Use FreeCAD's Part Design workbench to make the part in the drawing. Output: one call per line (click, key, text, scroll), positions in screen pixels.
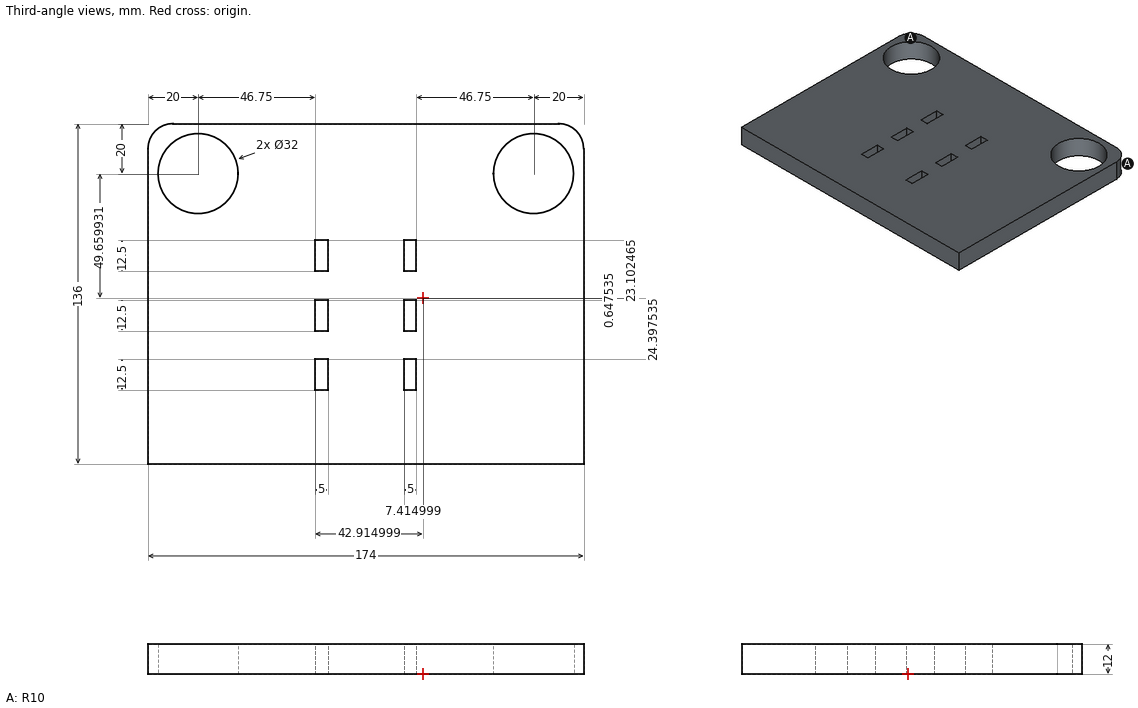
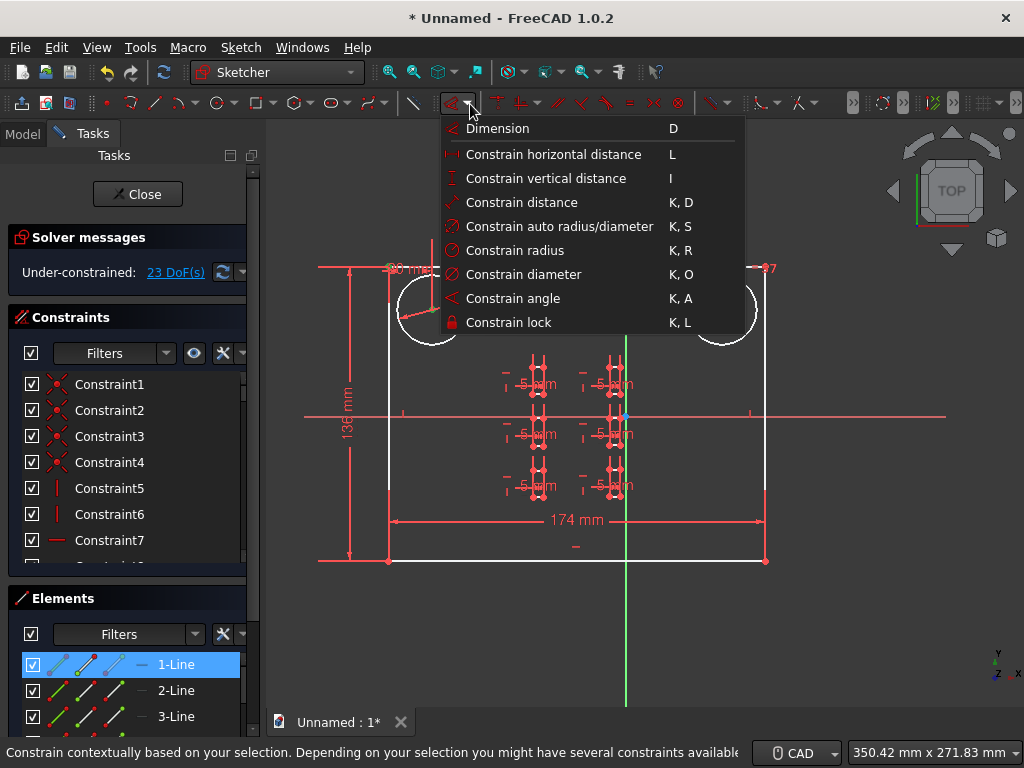
click(593, 178)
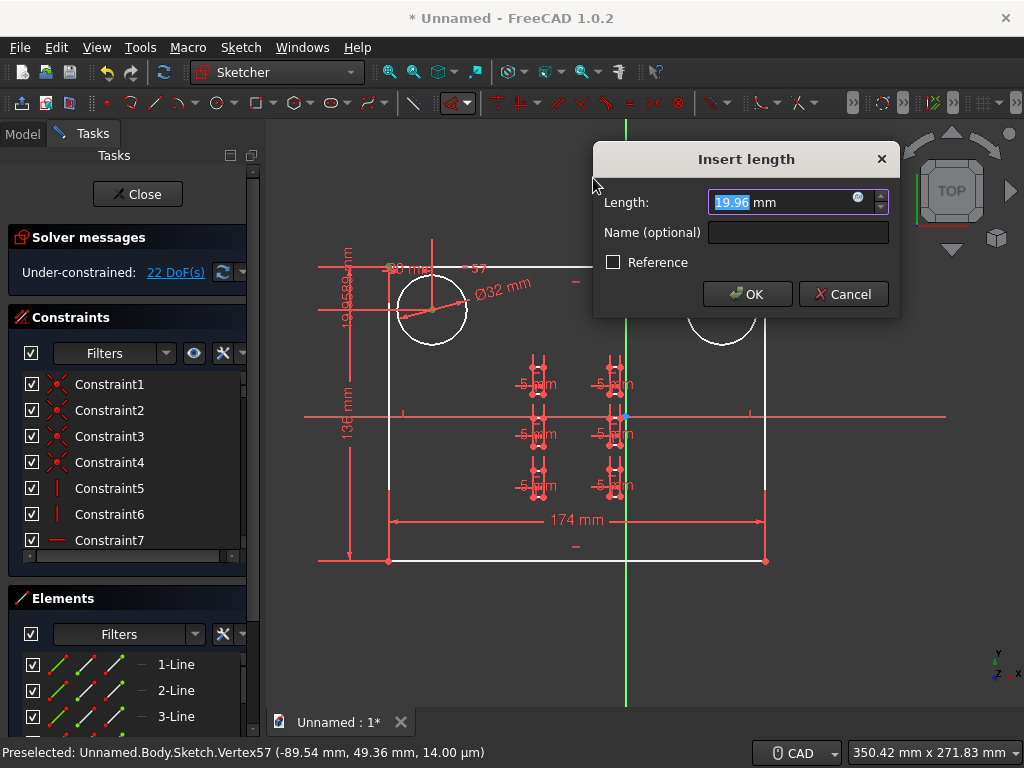
text(20)
key(Return)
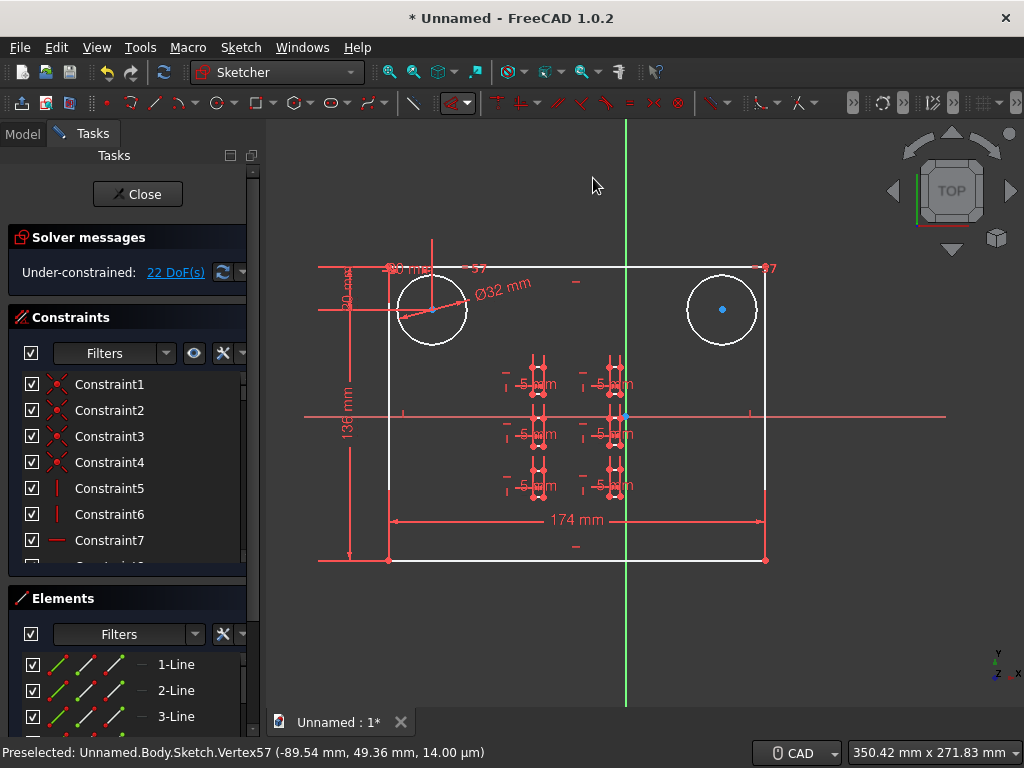
scroll(765, 267, up, 4)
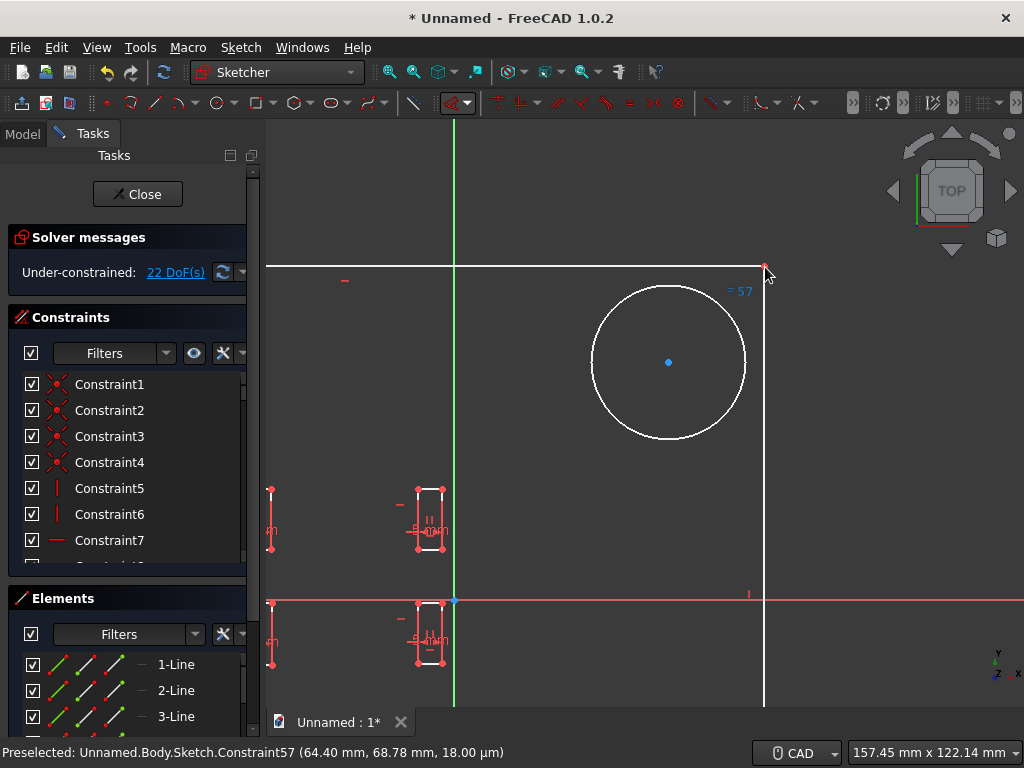
click(764, 266)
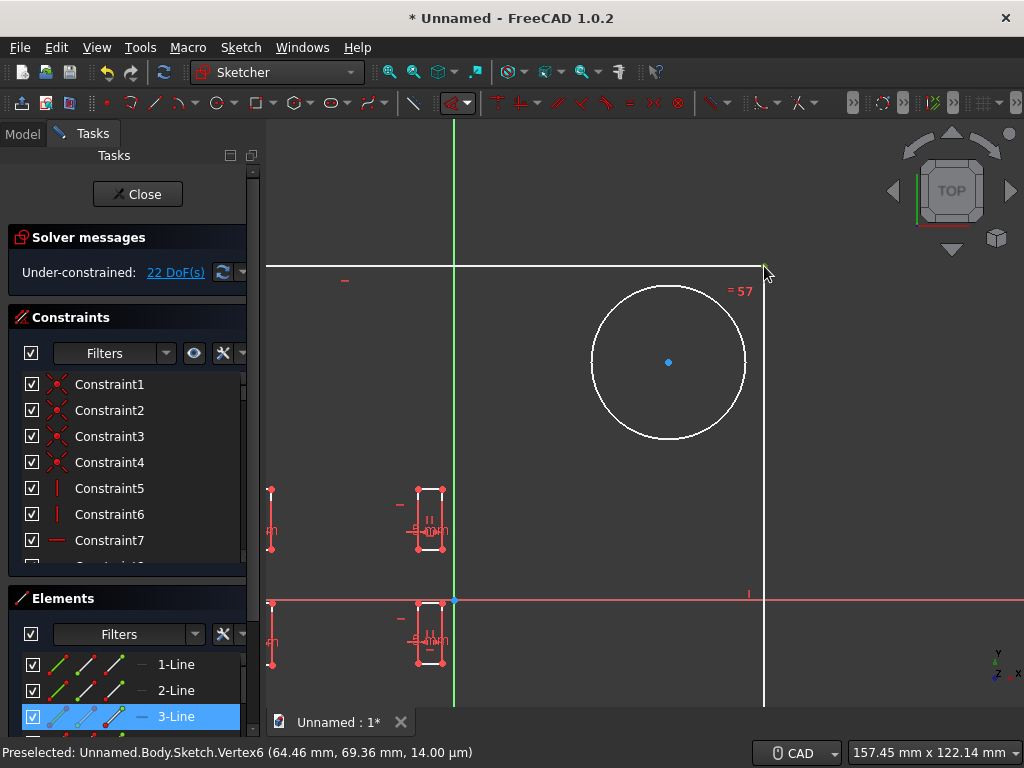
click(668, 362)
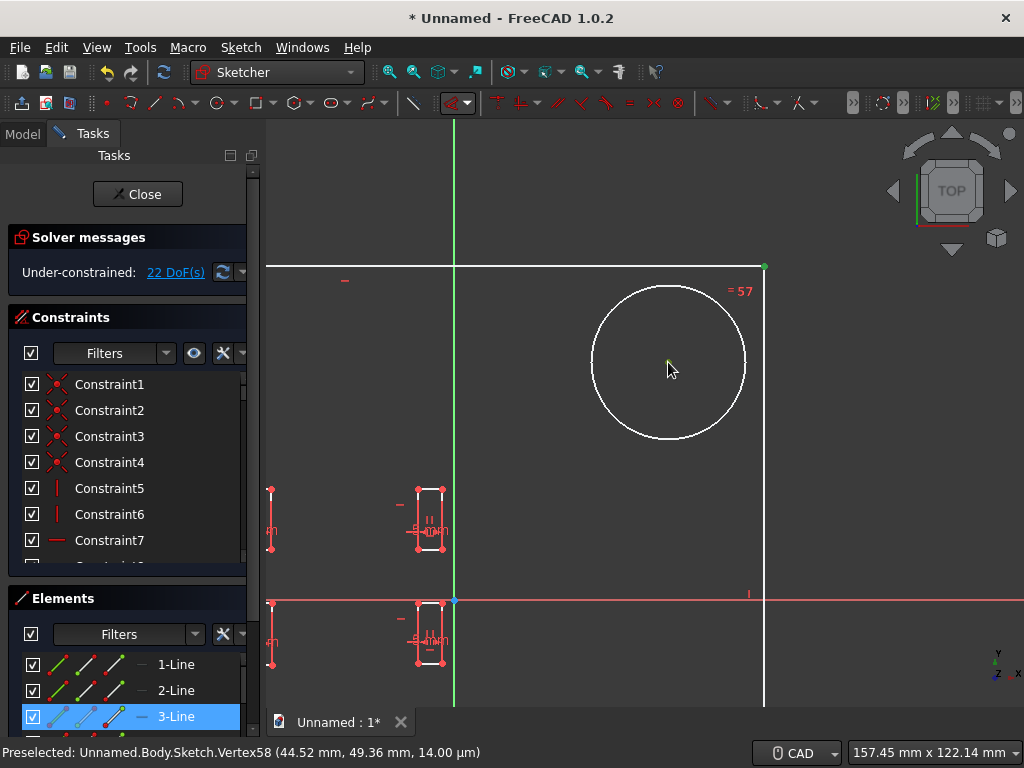
key(l)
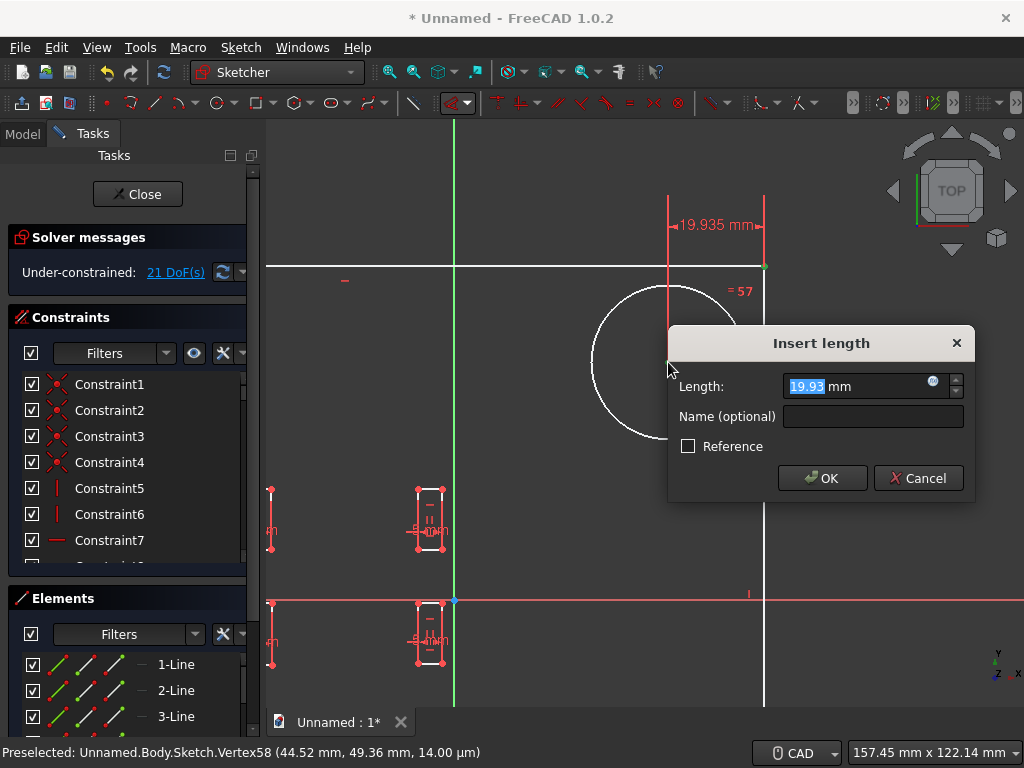
text(20)
key(Return)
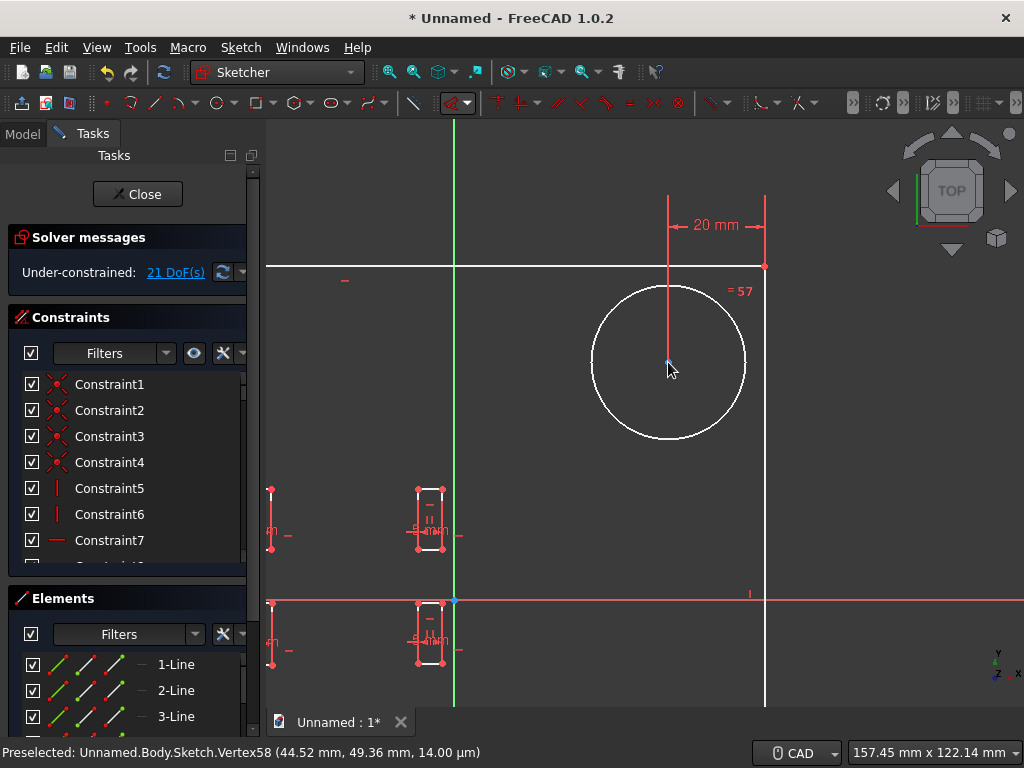
click(765, 266)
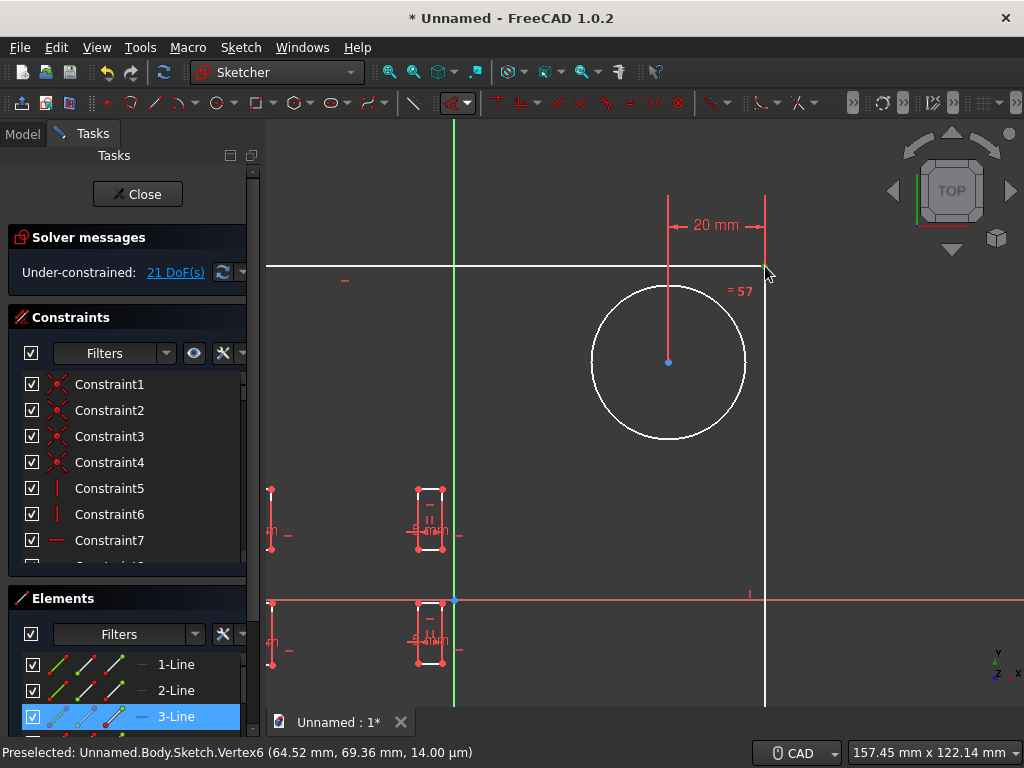
click(668, 362)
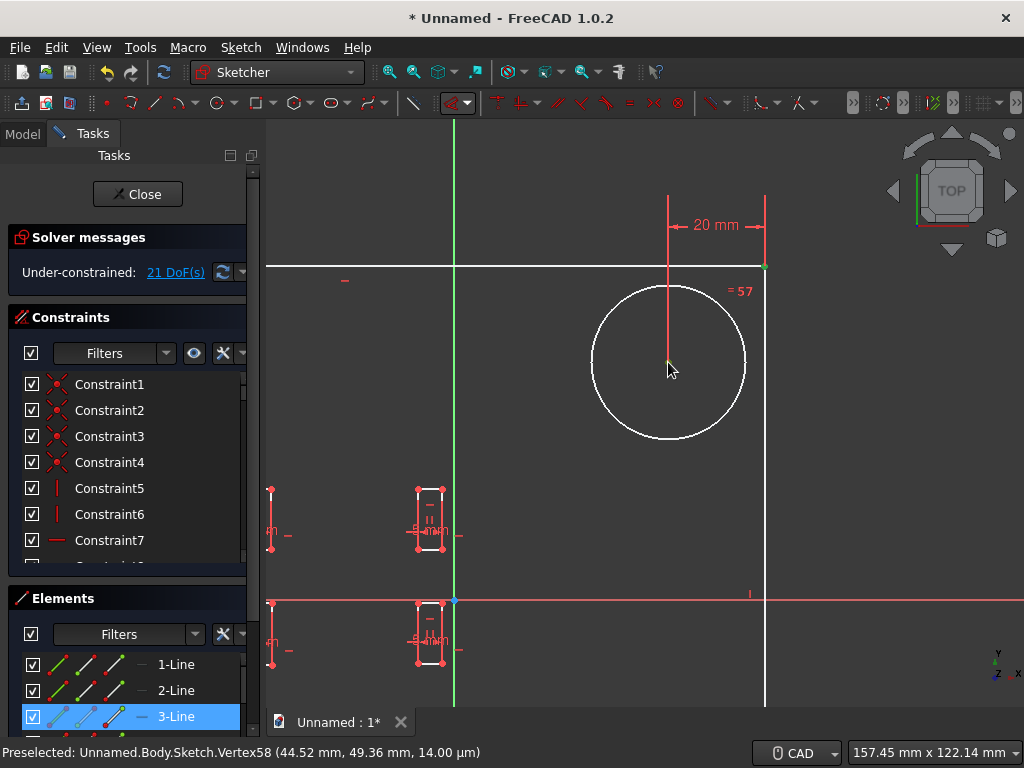
key(i)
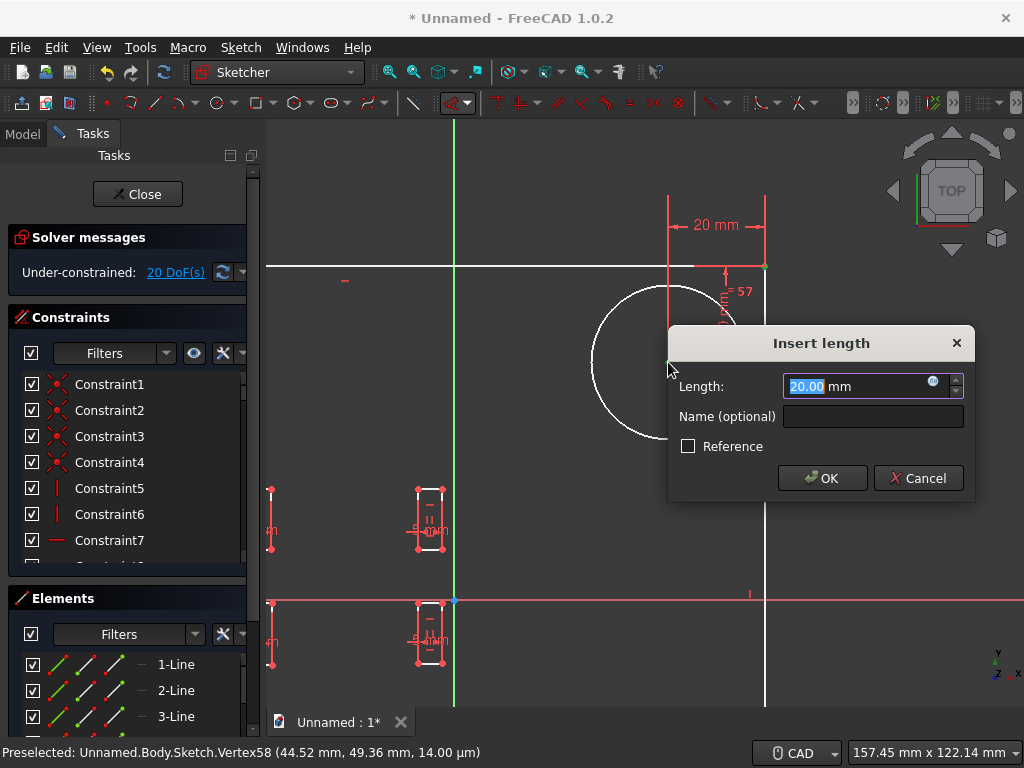
text(20)
key(Return)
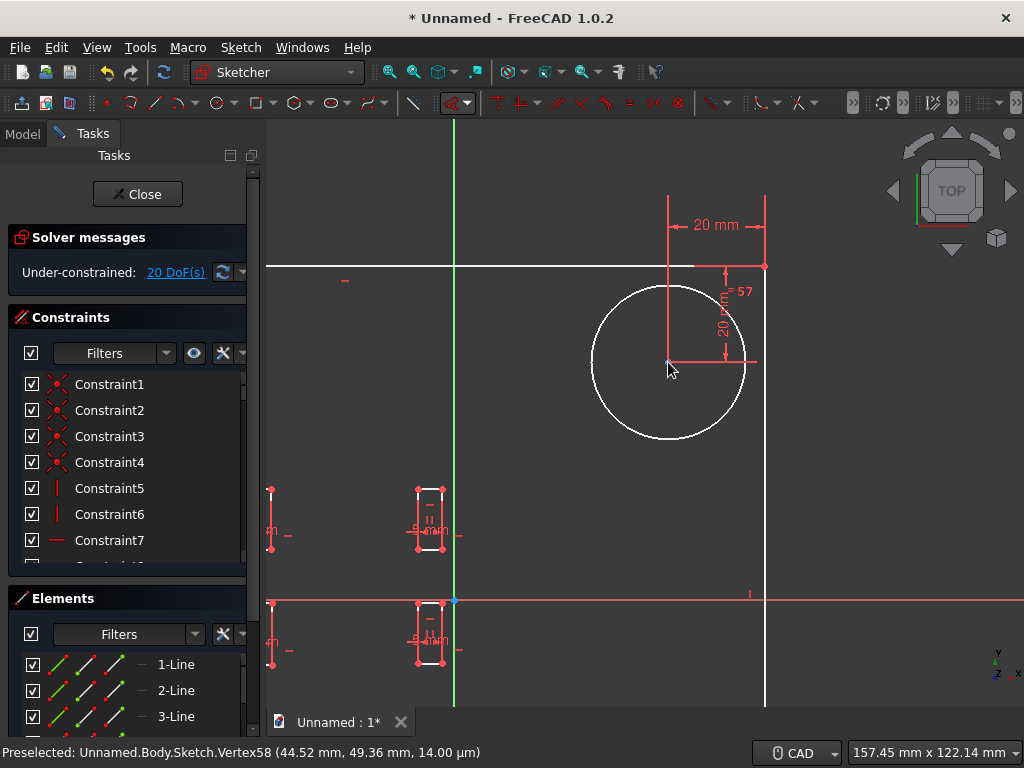
scroll(765, 267, down, 4)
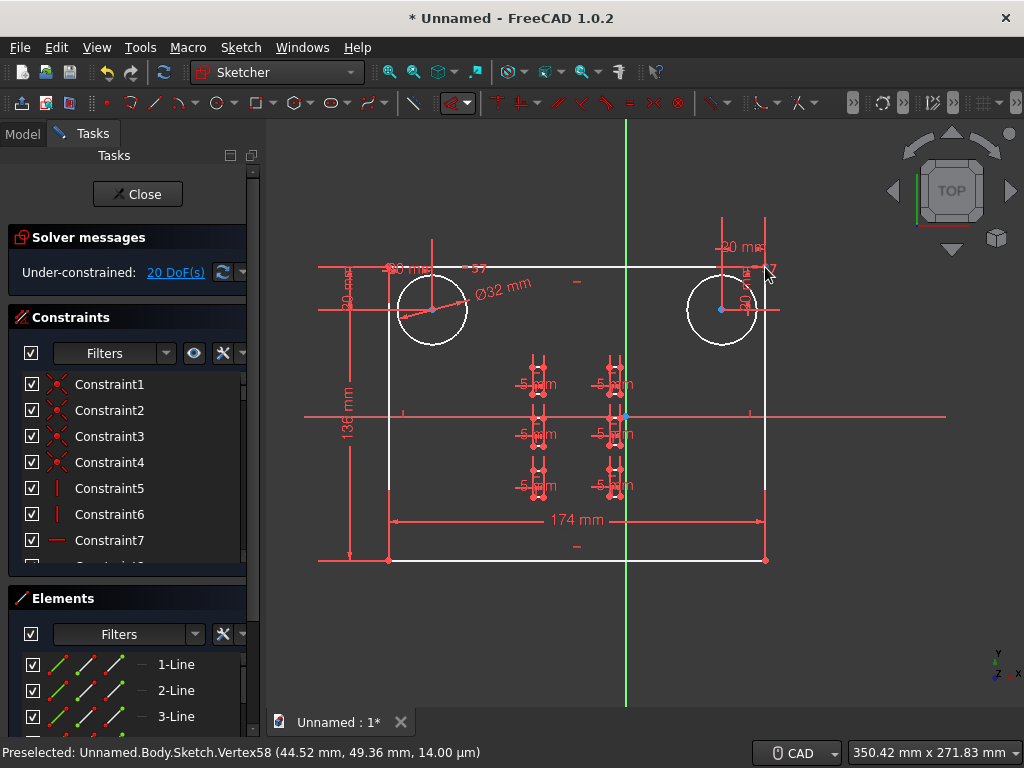
scroll(533, 479, up, 3)